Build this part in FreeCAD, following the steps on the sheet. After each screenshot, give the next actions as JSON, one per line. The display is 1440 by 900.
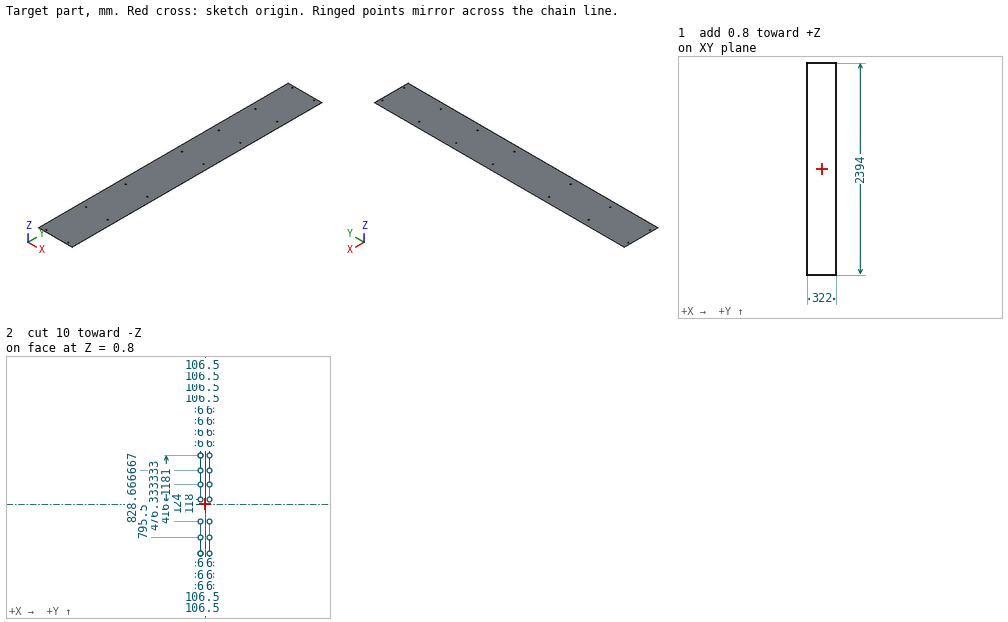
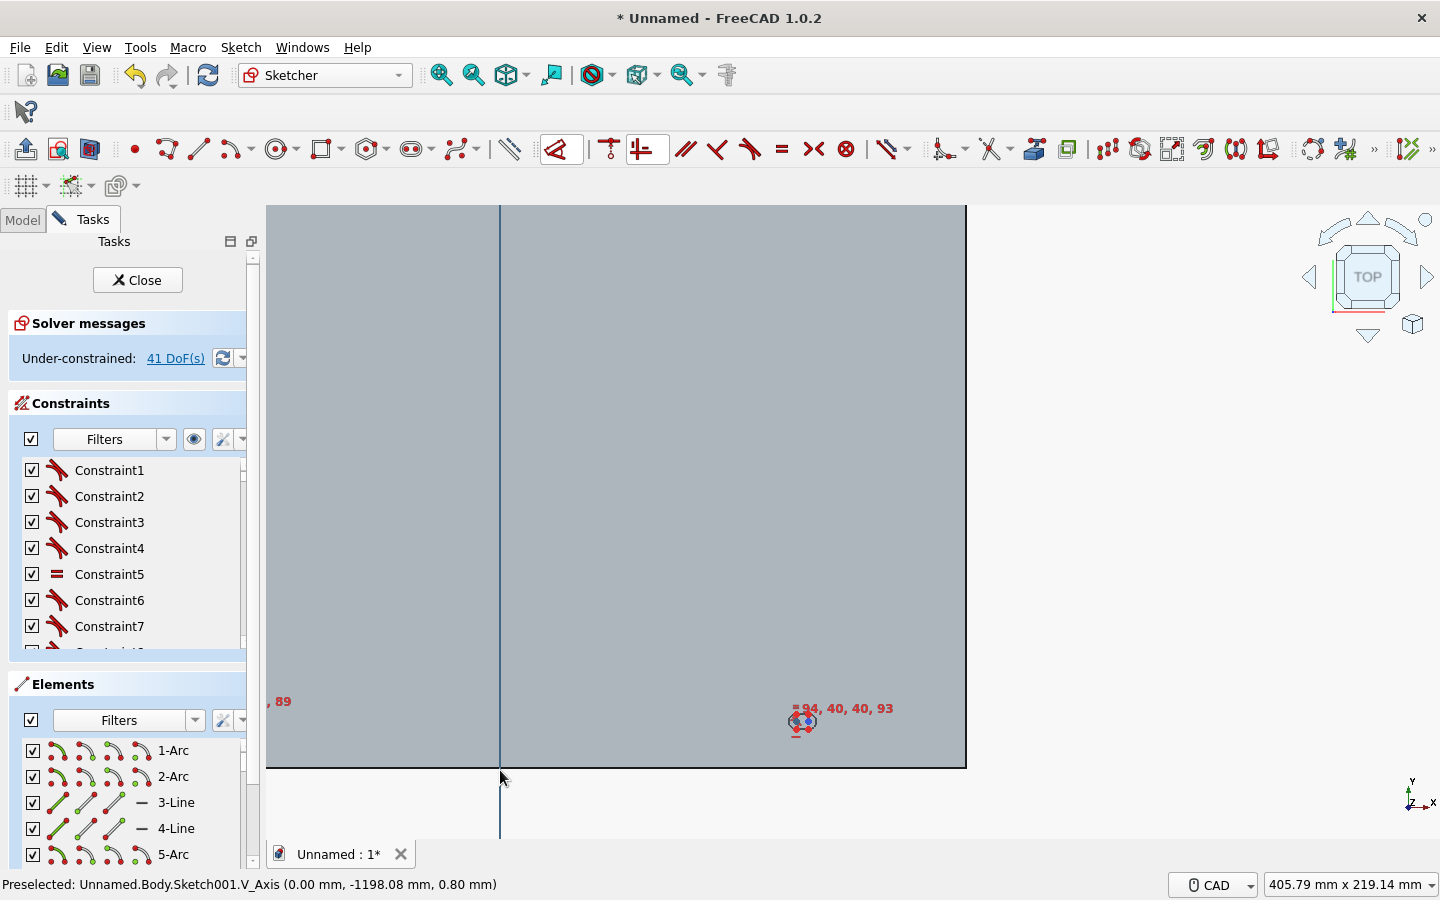
{"action": "key", "text": "s"}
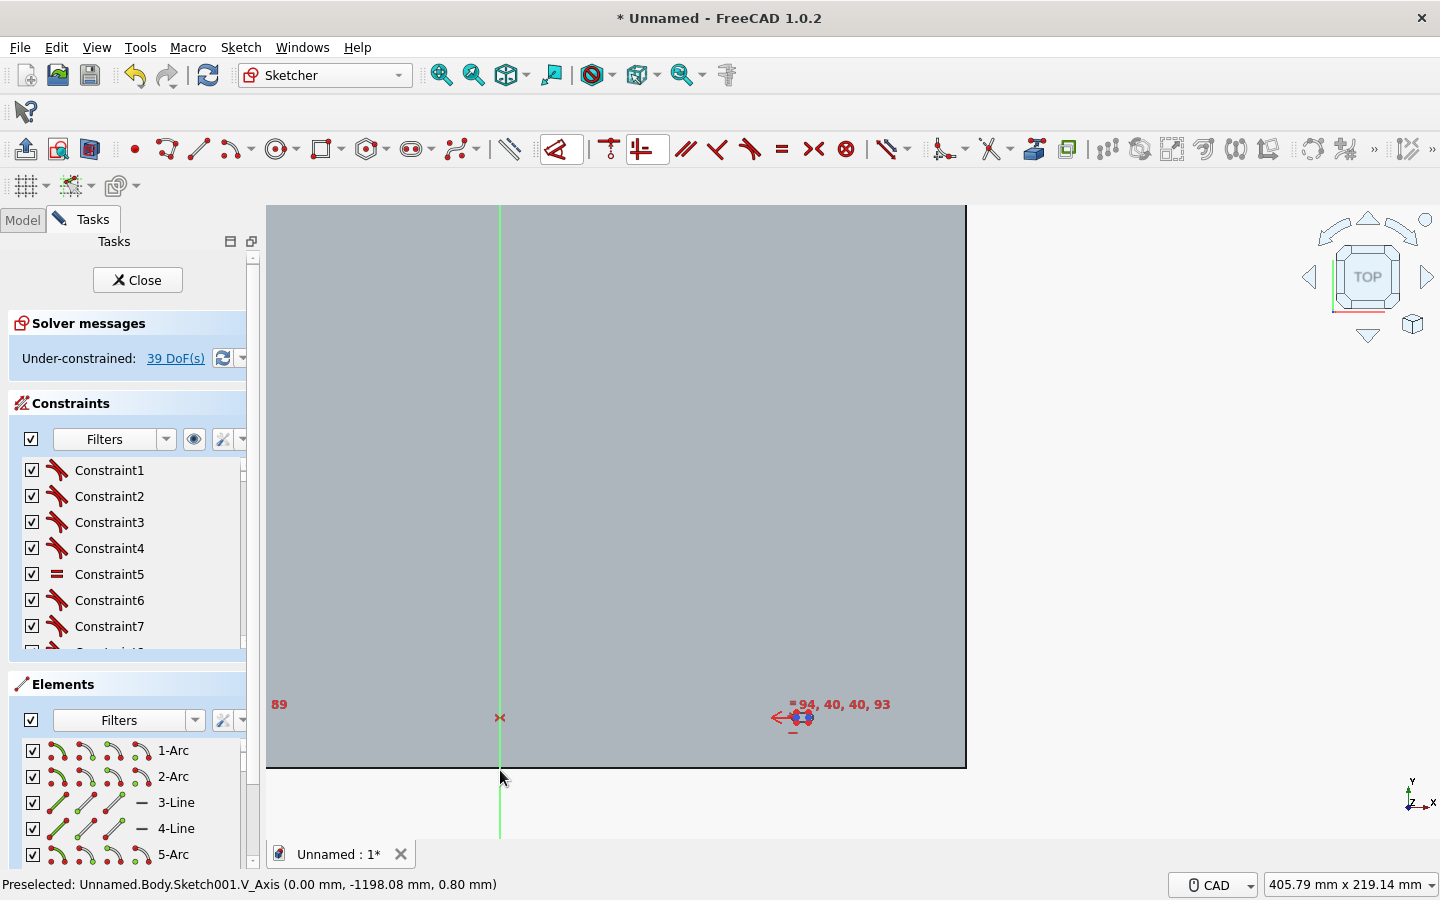
{"action": "scroll", "coordinate": [803, 730], "scroll_direction": "down", "scroll_amount": 14}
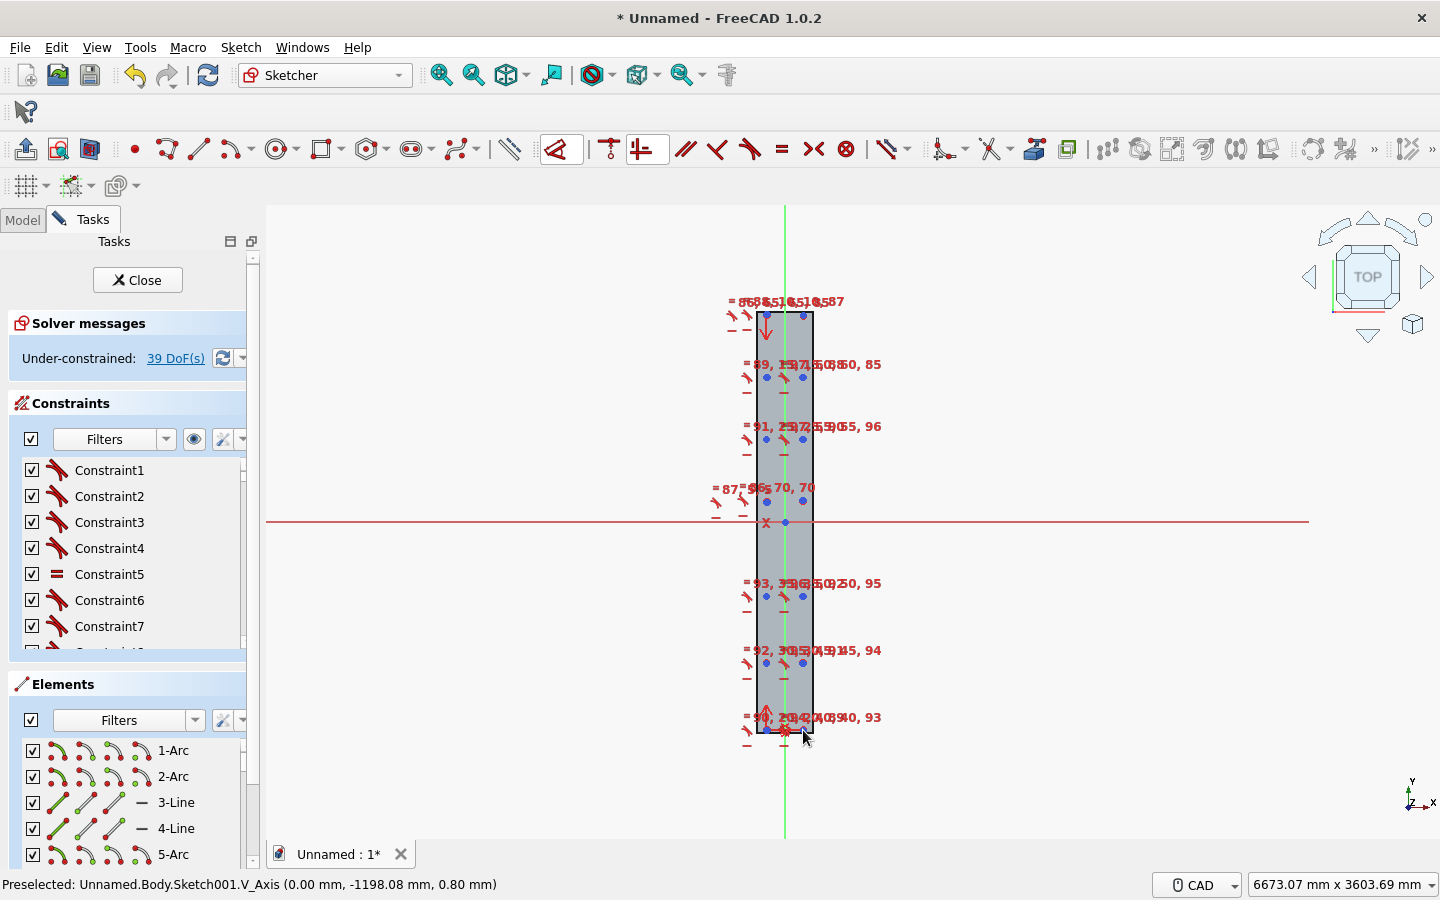
{"action": "scroll", "coordinate": [767, 663], "scroll_direction": "up", "scroll_amount": 14}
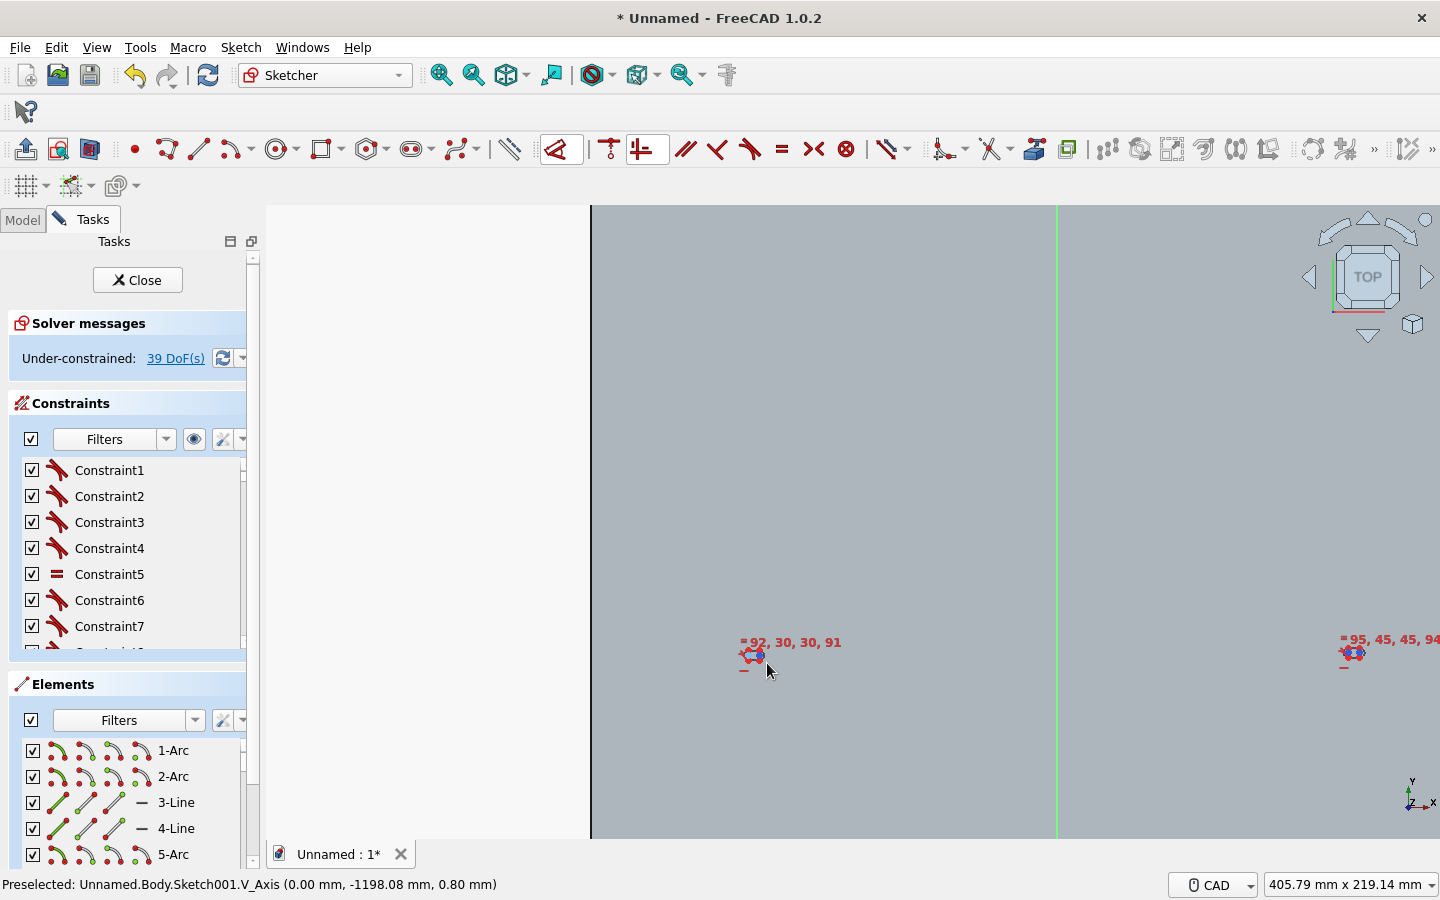
{"action": "left_click", "coordinate": [759, 655]}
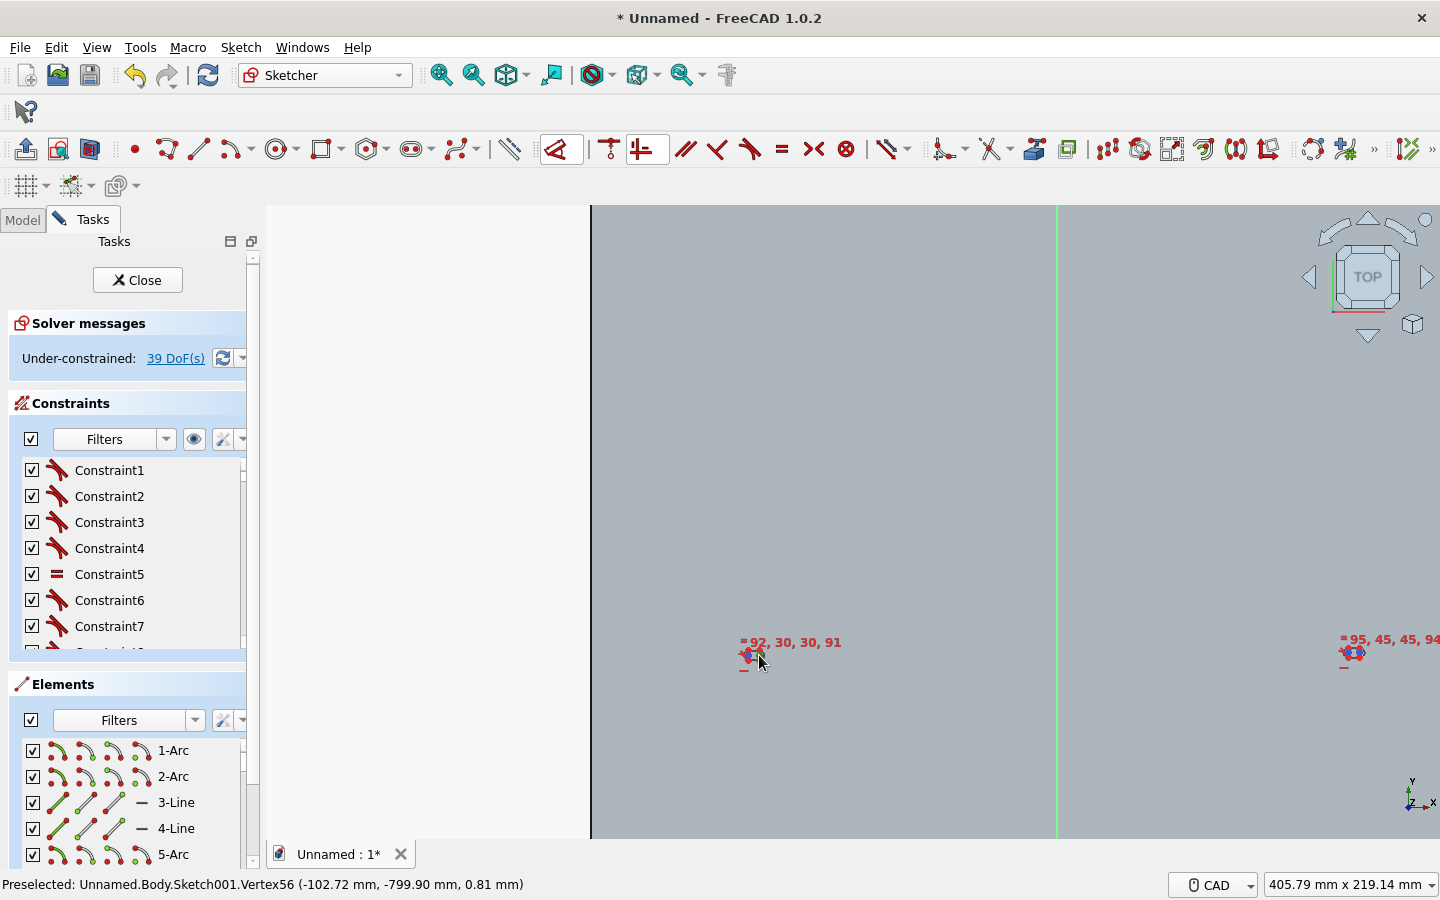
{"action": "scroll", "coordinate": [767, 663], "scroll_direction": "down", "scroll_amount": 14}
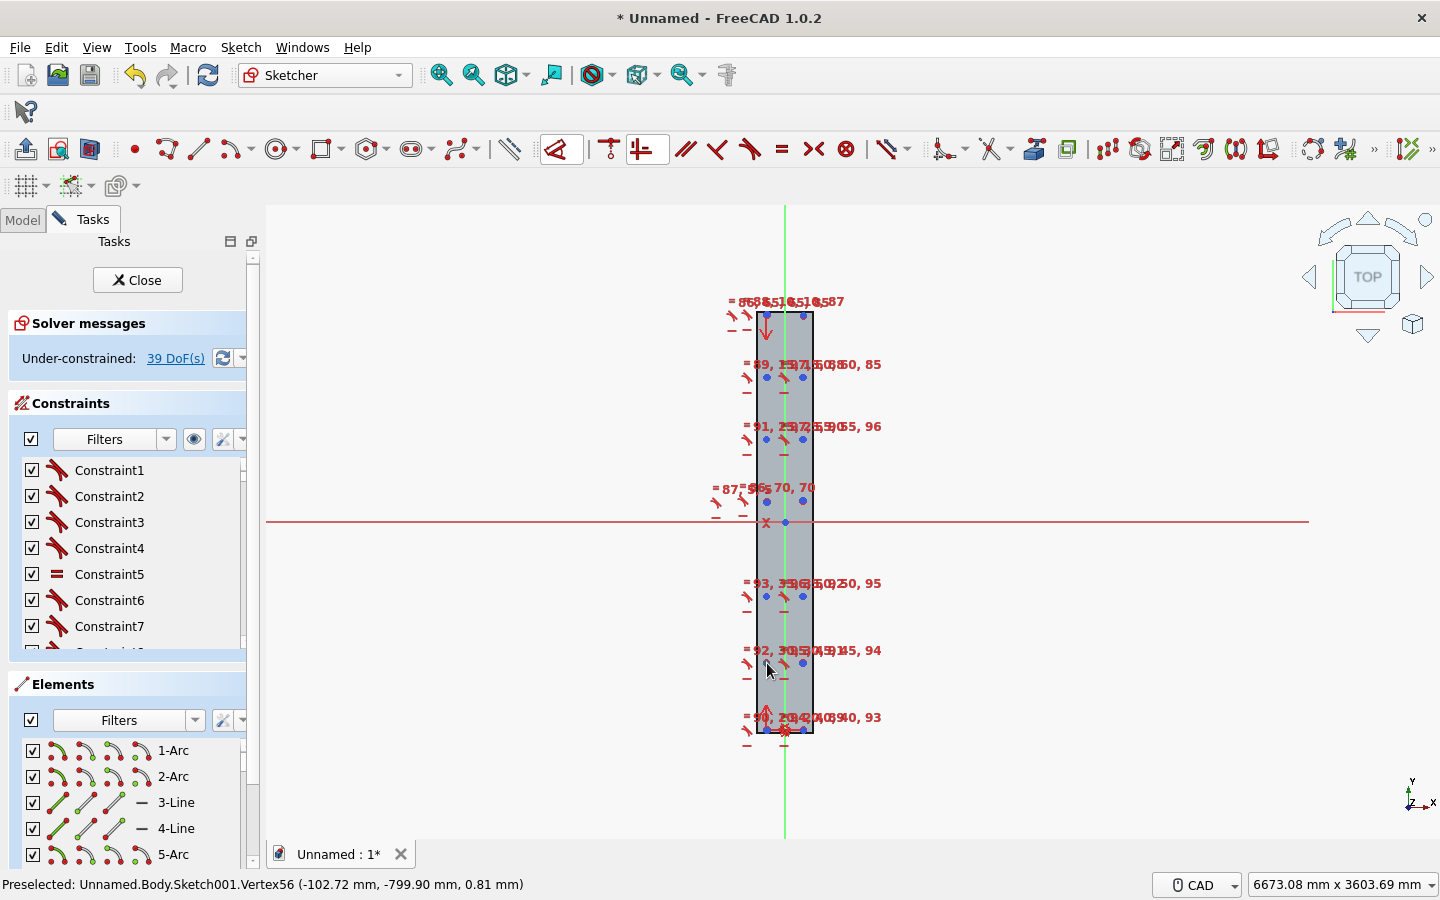
{"action": "scroll", "coordinate": [803, 663], "scroll_direction": "up", "scroll_amount": 14}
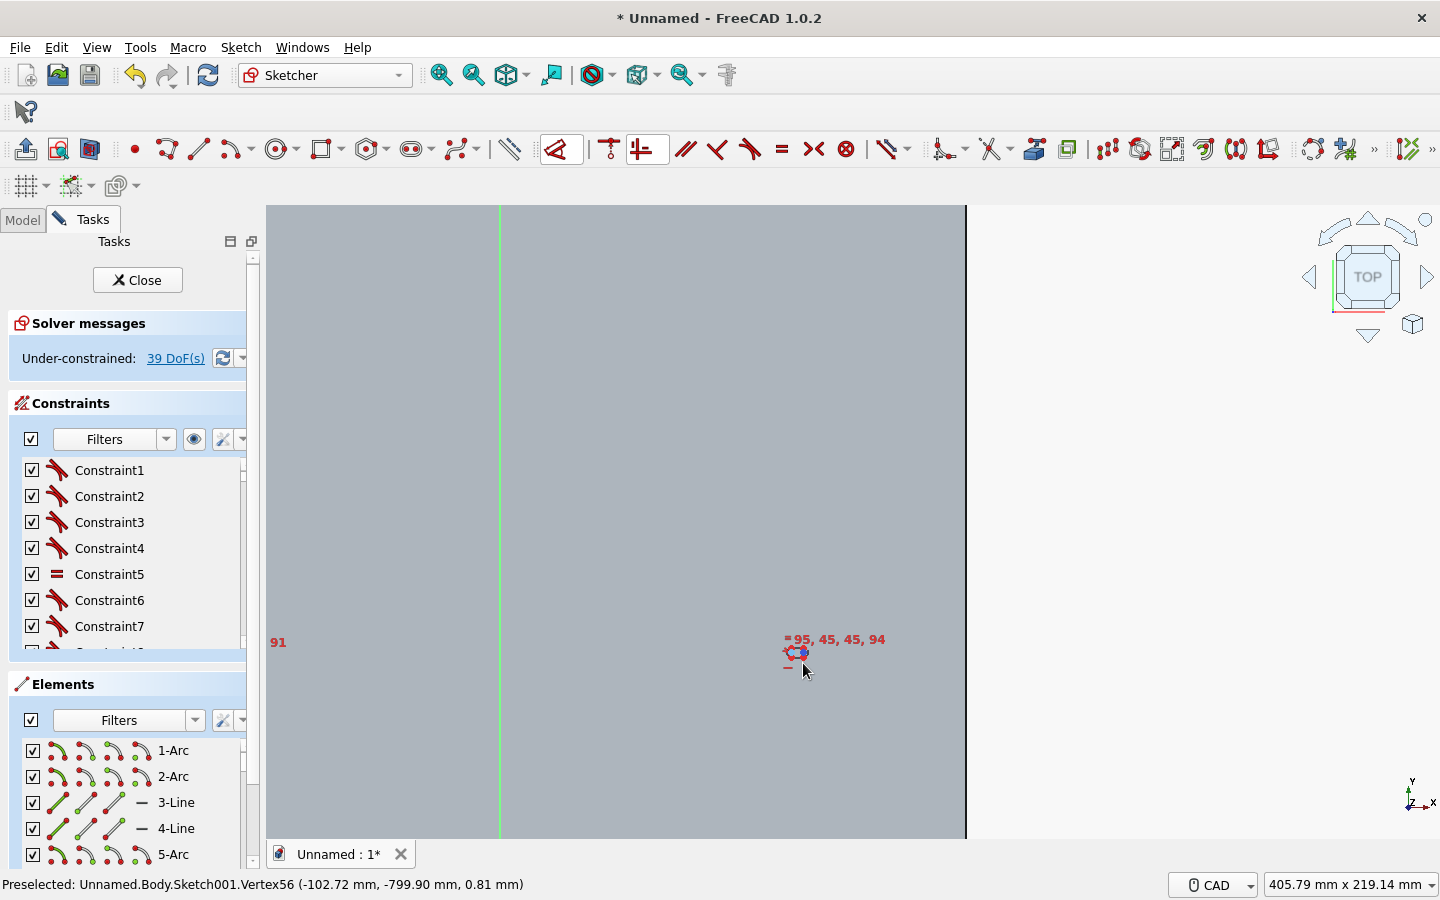
{"action": "left_click", "coordinate": [792, 653]}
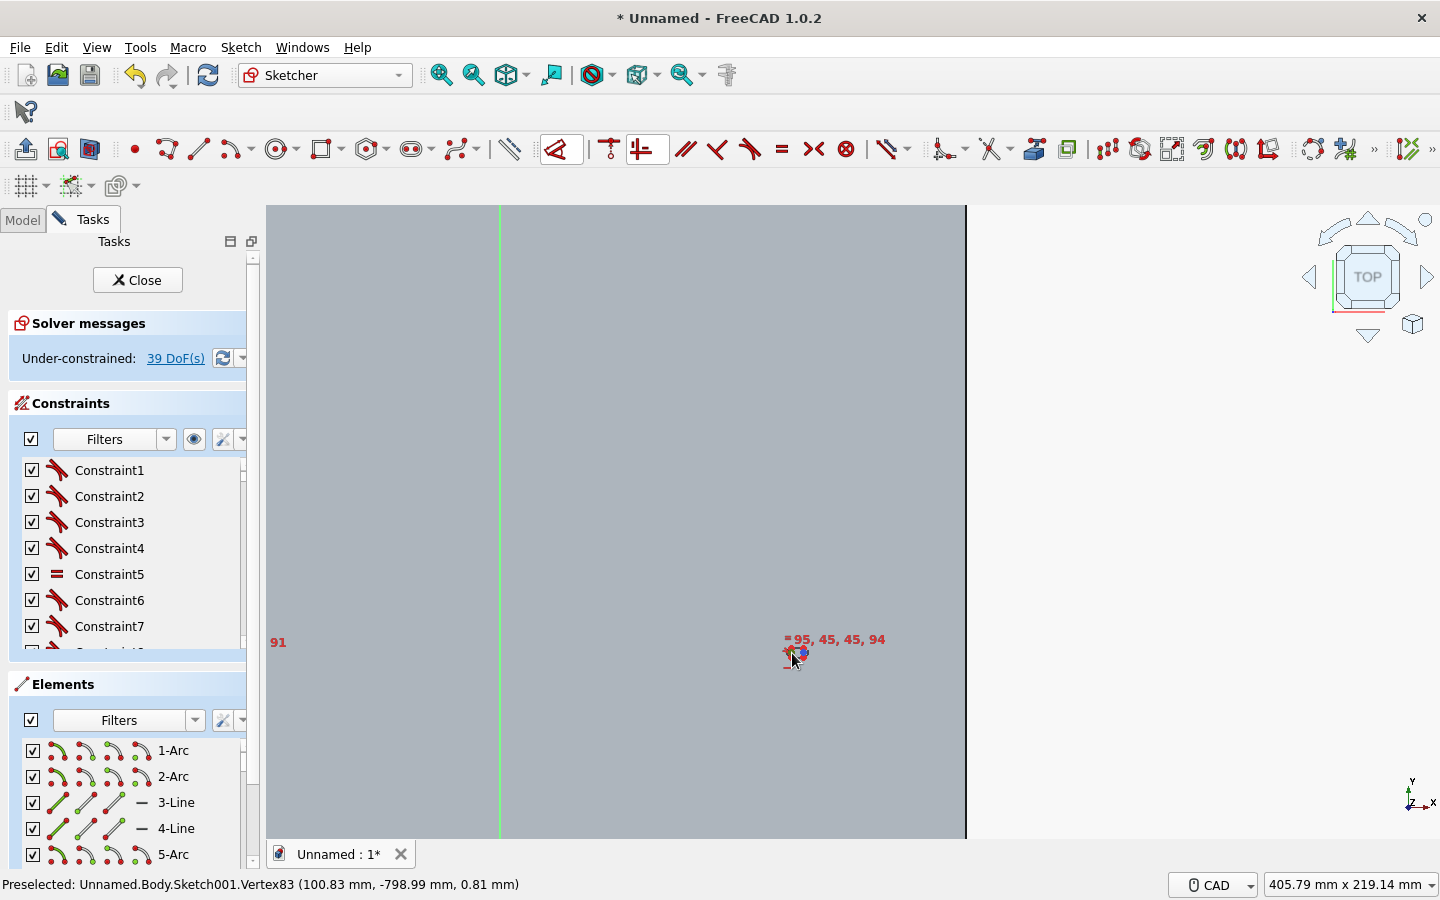
{"action": "left_click", "coordinate": [500, 770]}